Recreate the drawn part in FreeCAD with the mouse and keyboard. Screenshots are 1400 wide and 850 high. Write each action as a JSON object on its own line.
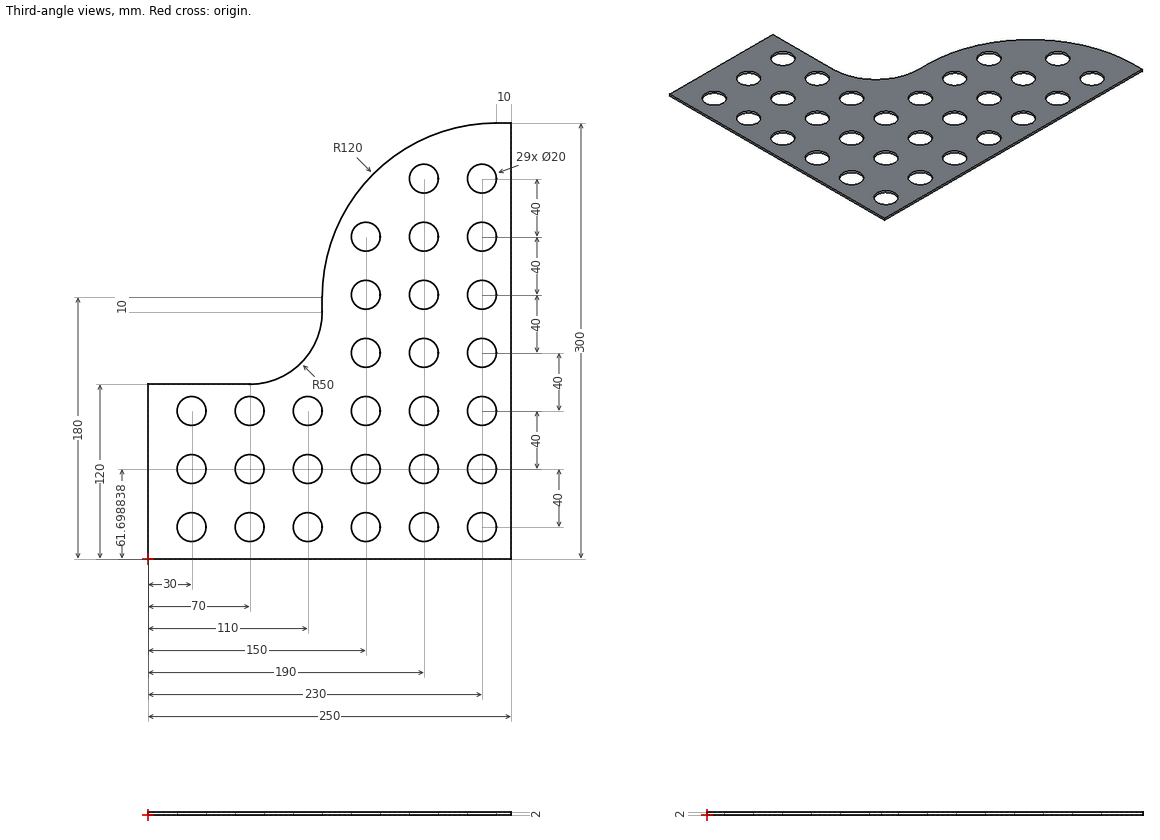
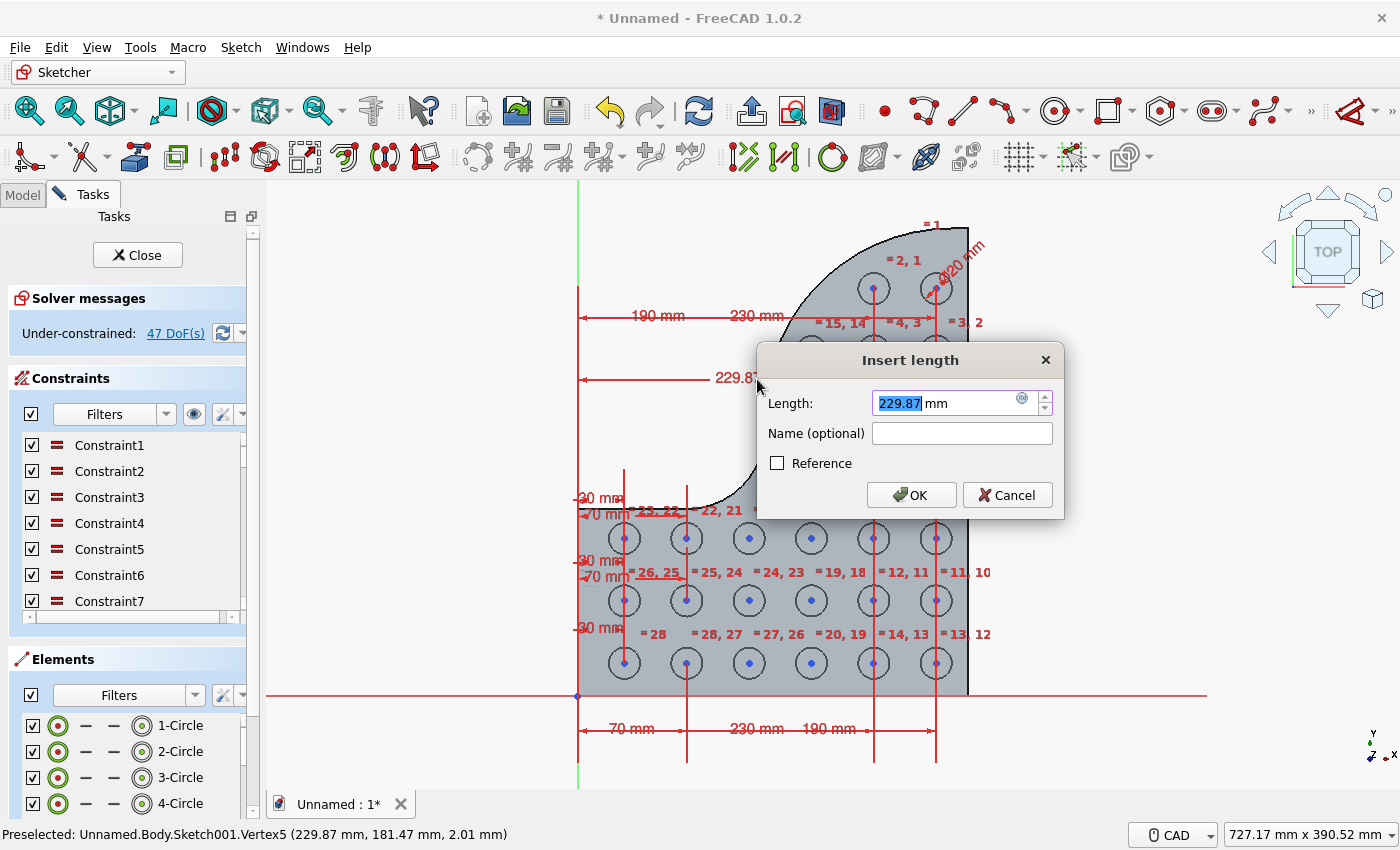
{"action": "type", "text": "230"}
{"action": "key", "text": "Return"}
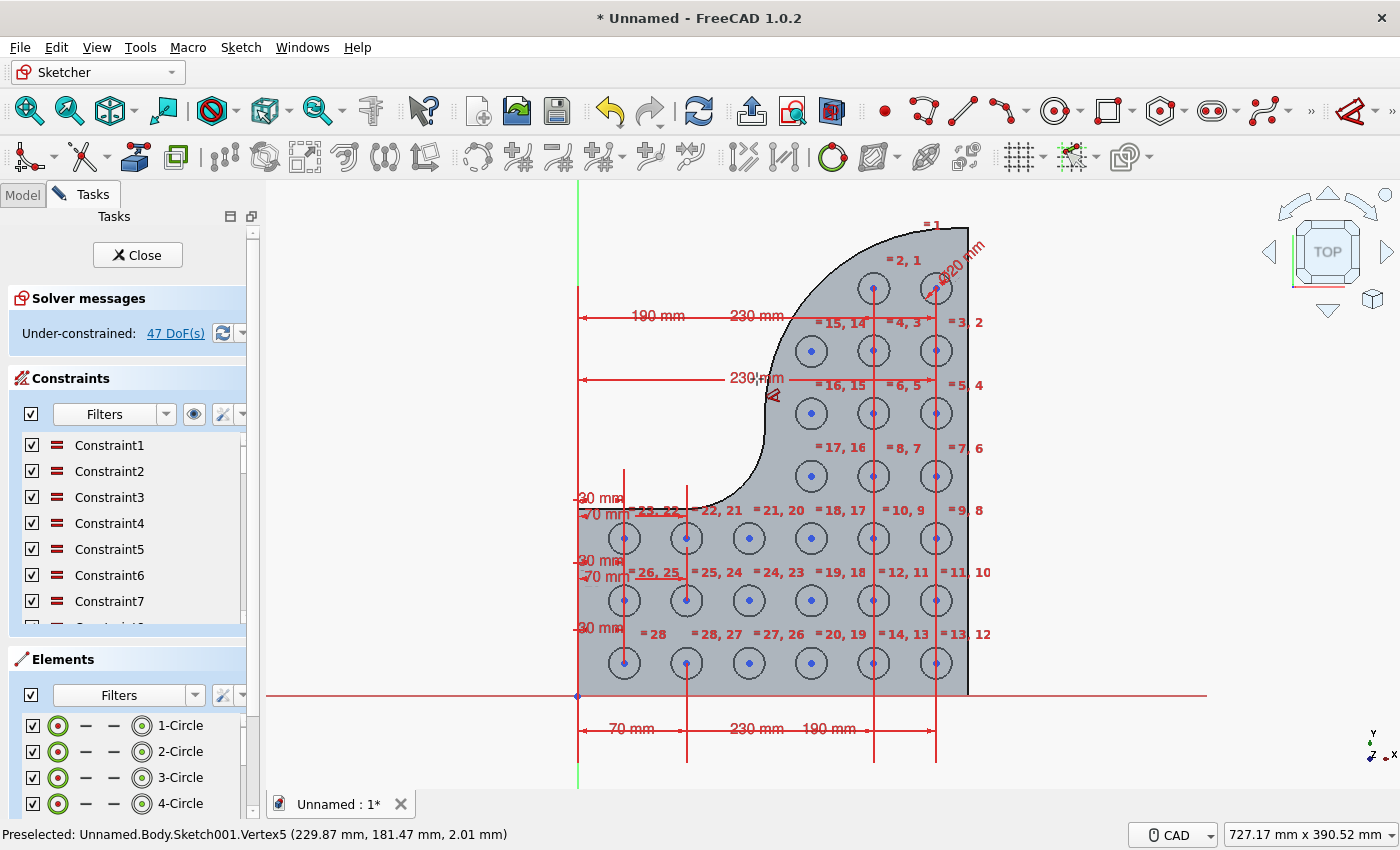
{"action": "left_click", "coordinate": [874, 413]}
{"action": "left_click", "coordinate": [658, 379]}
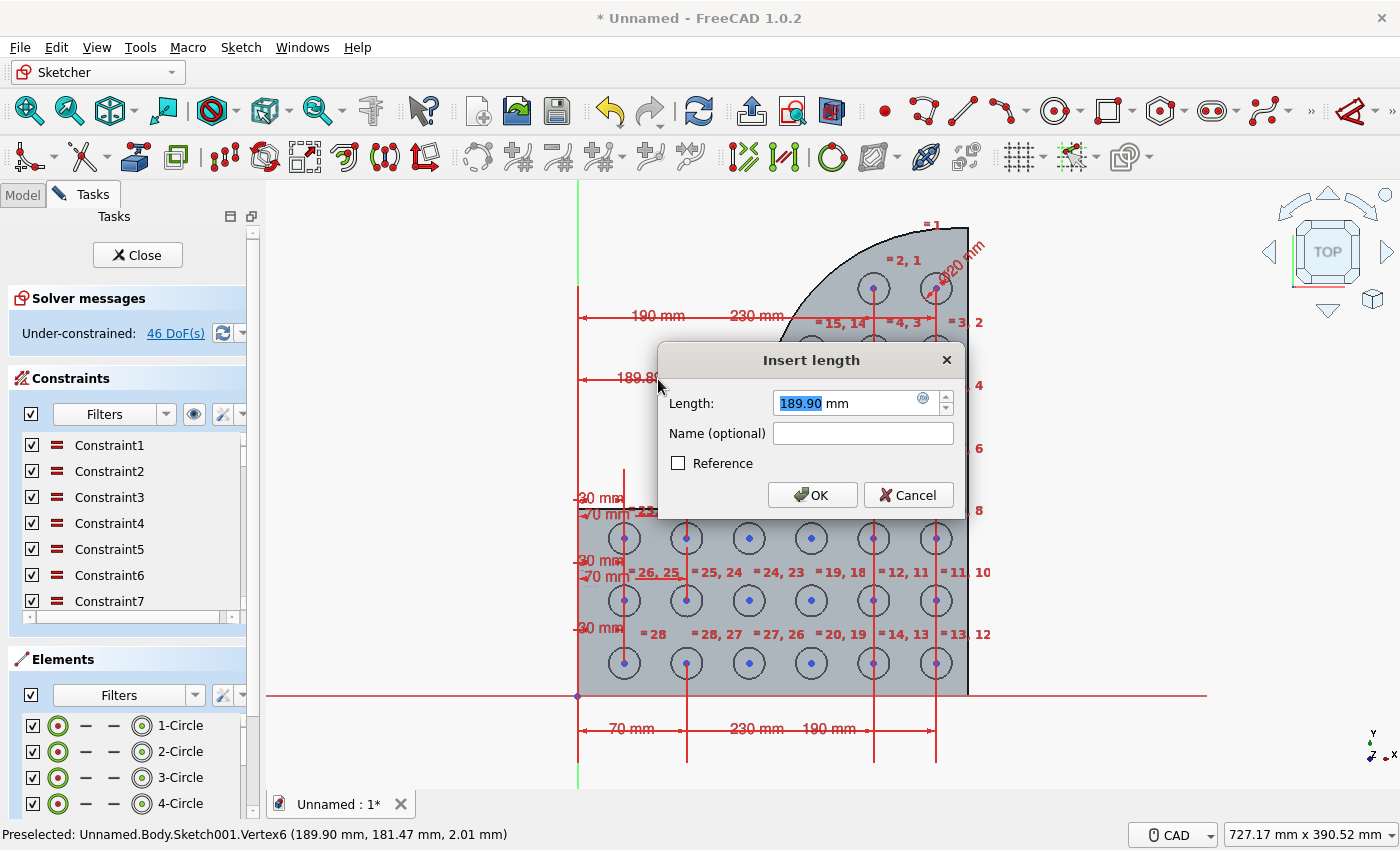
{"action": "type", "text": "190"}
{"action": "key", "text": "Return"}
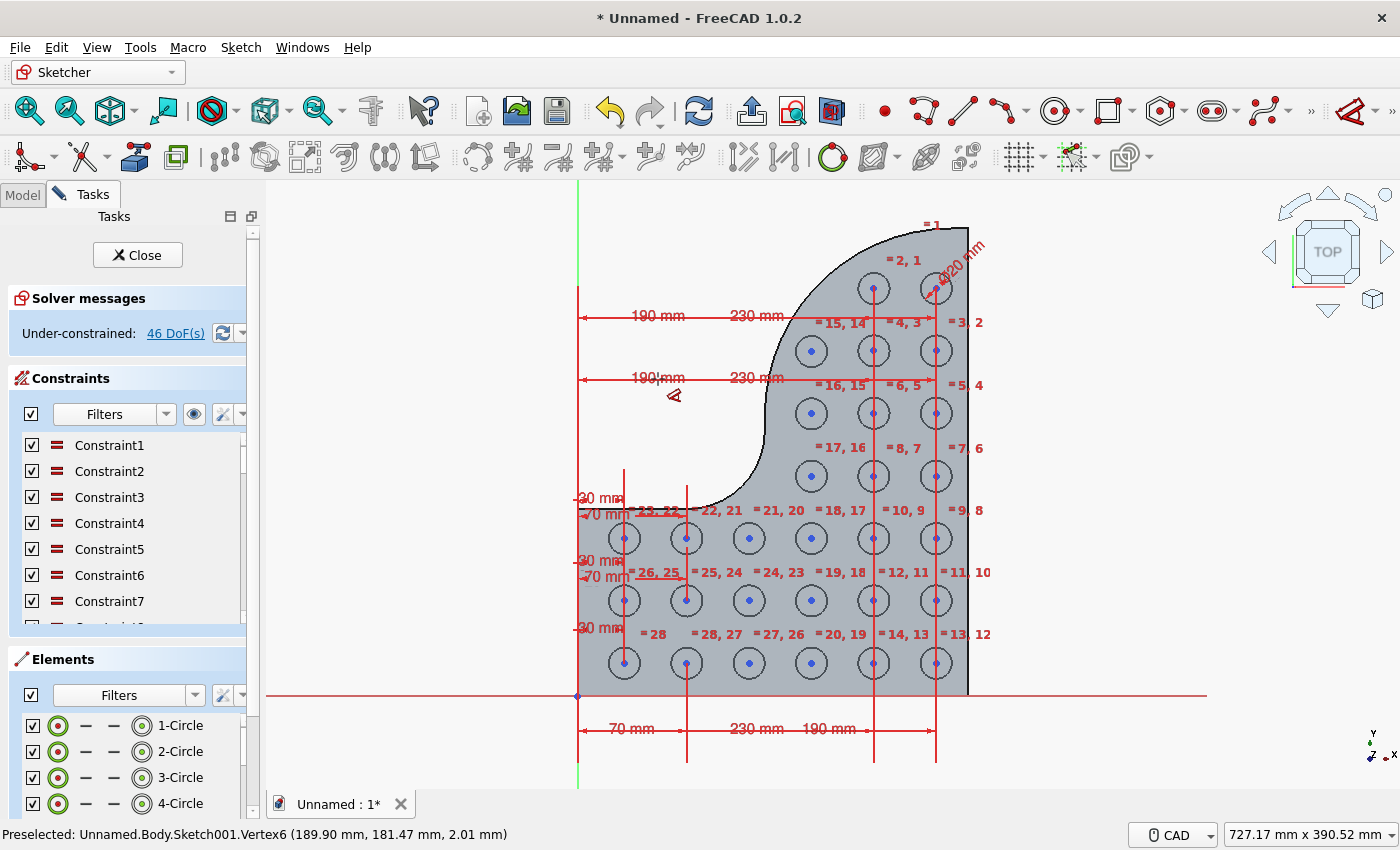
{"action": "left_click", "coordinate": [936, 476]}
{"action": "left_click", "coordinate": [757, 442]}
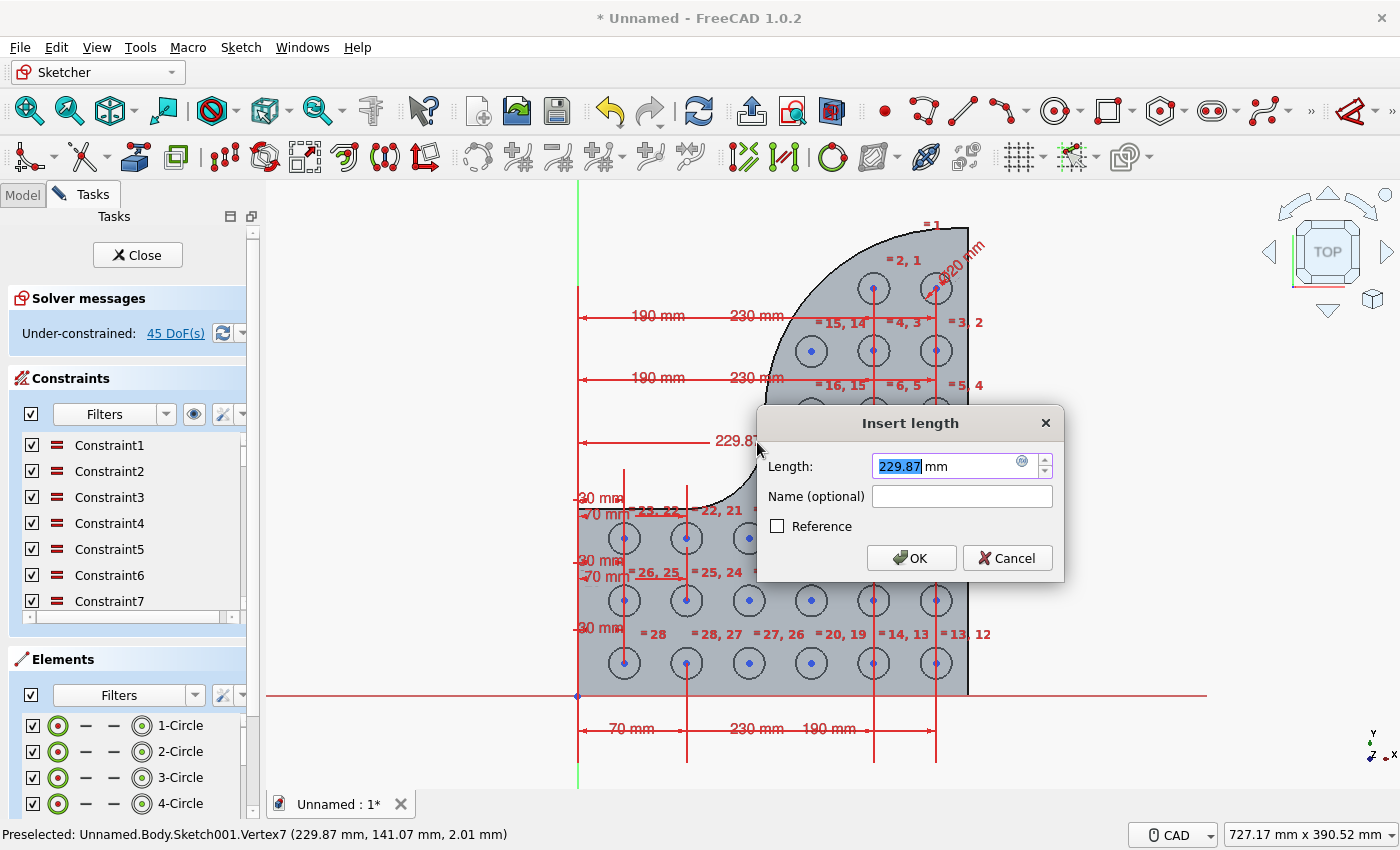
{"action": "type", "text": "230"}
{"action": "key", "text": "Return"}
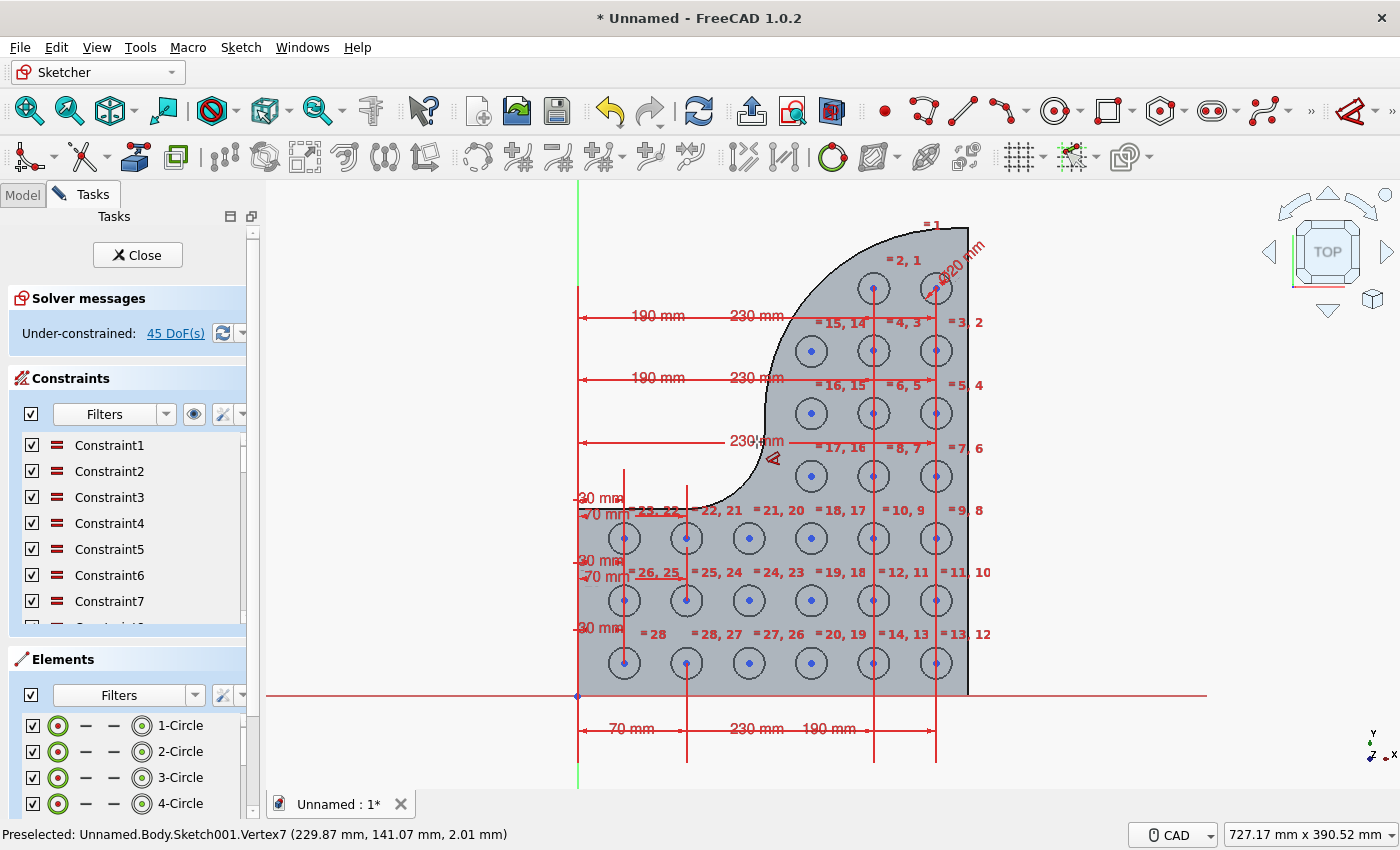
{"action": "left_click", "coordinate": [874, 476]}
{"action": "left_click", "coordinate": [658, 442]}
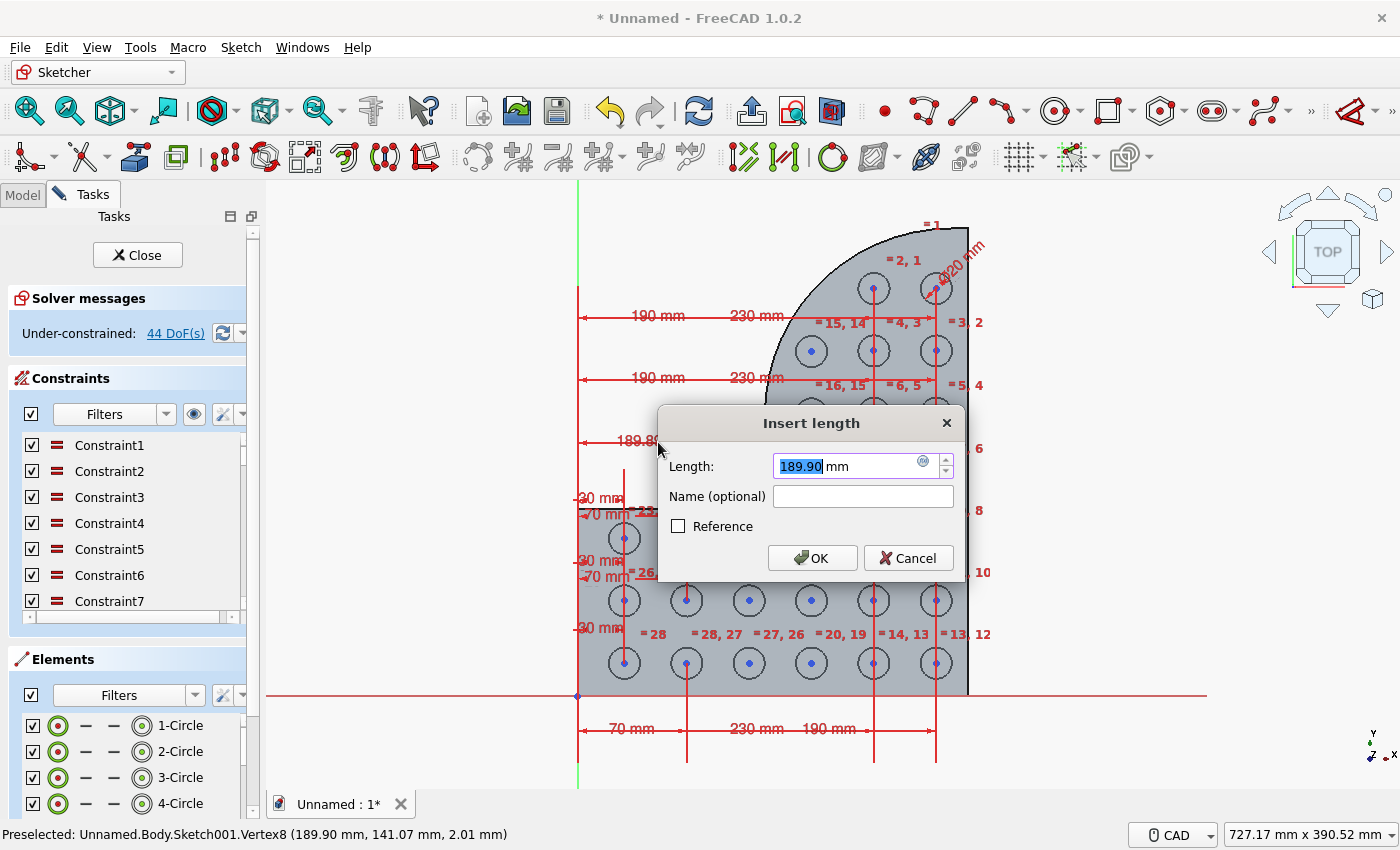
{"action": "type", "text": "190"}
{"action": "key", "text": "Return"}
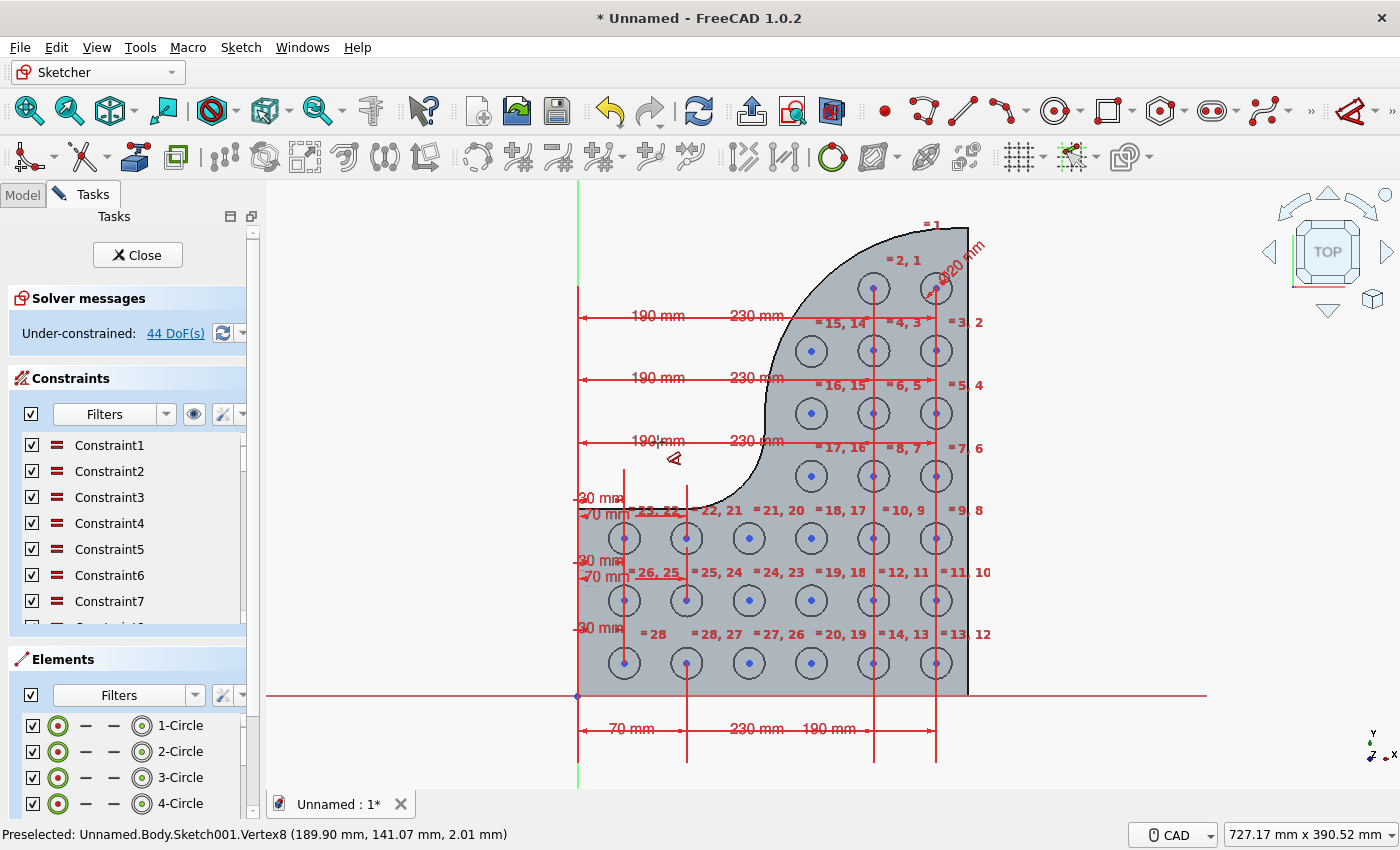
{"action": "left_click", "coordinate": [936, 539]}
{"action": "left_click", "coordinate": [757, 505]}